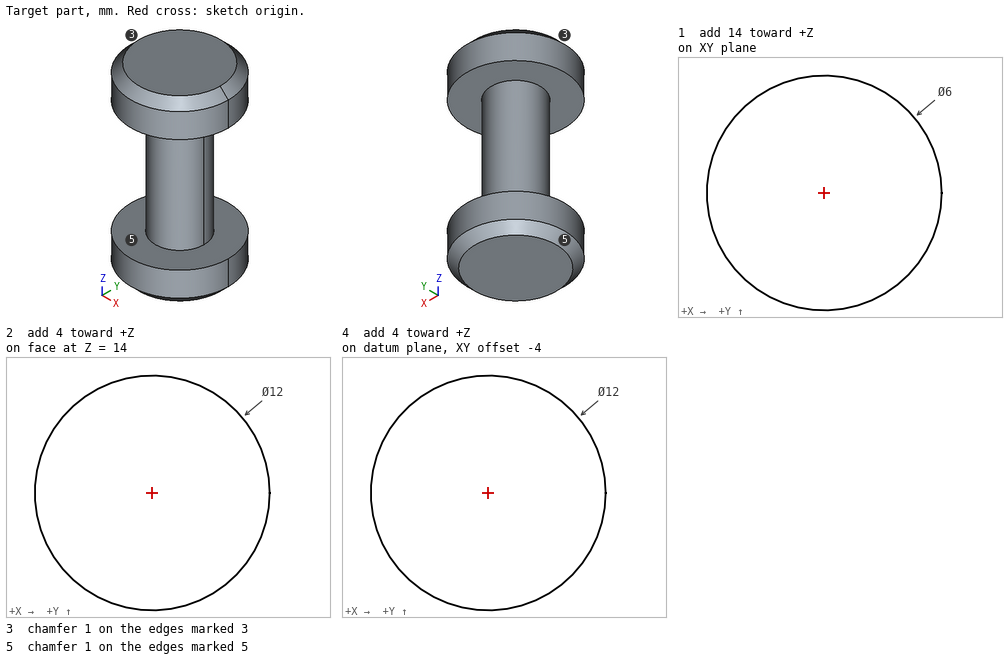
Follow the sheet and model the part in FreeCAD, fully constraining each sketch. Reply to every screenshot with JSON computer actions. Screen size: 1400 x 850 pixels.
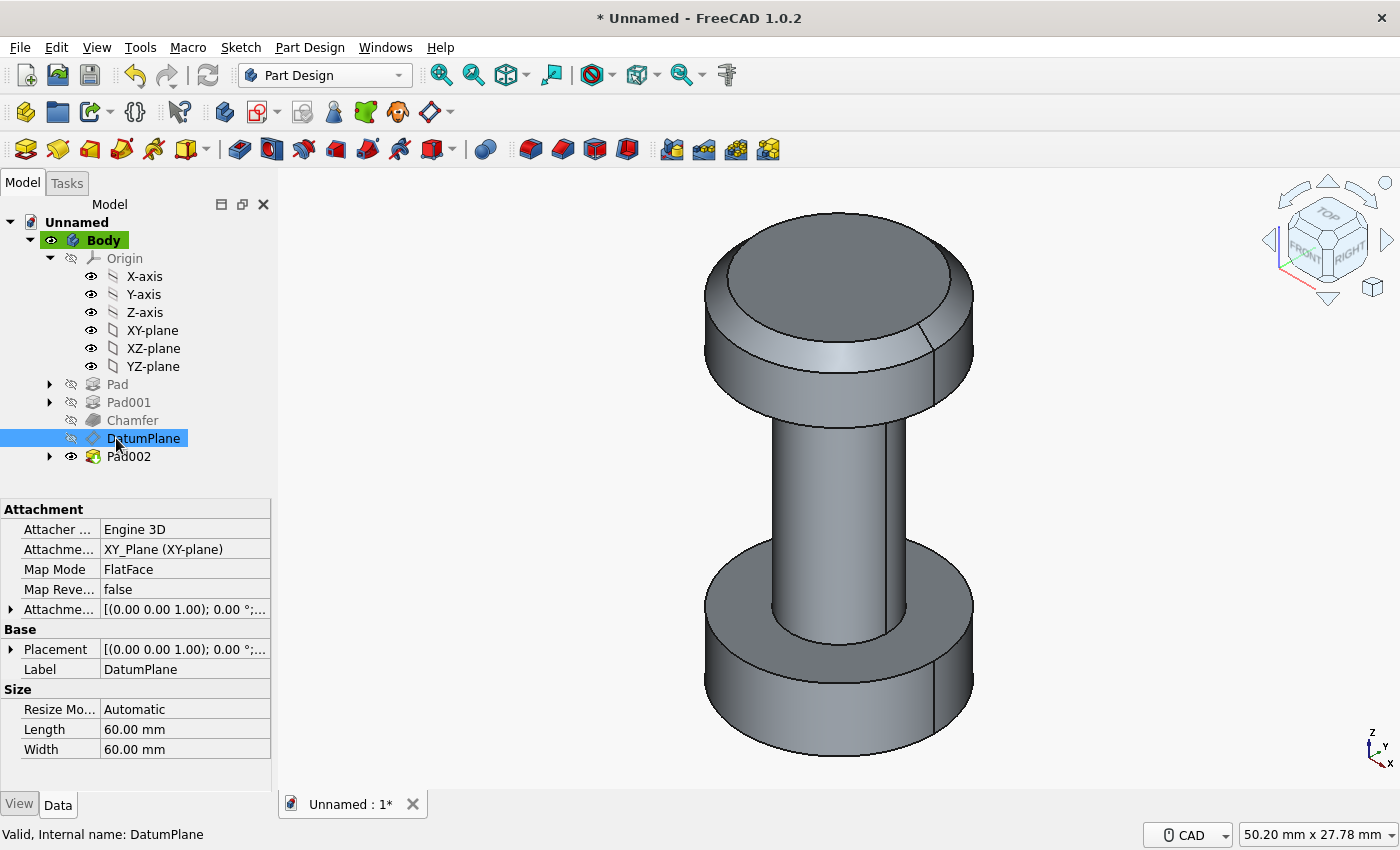
{"action": "key", "text": "2"}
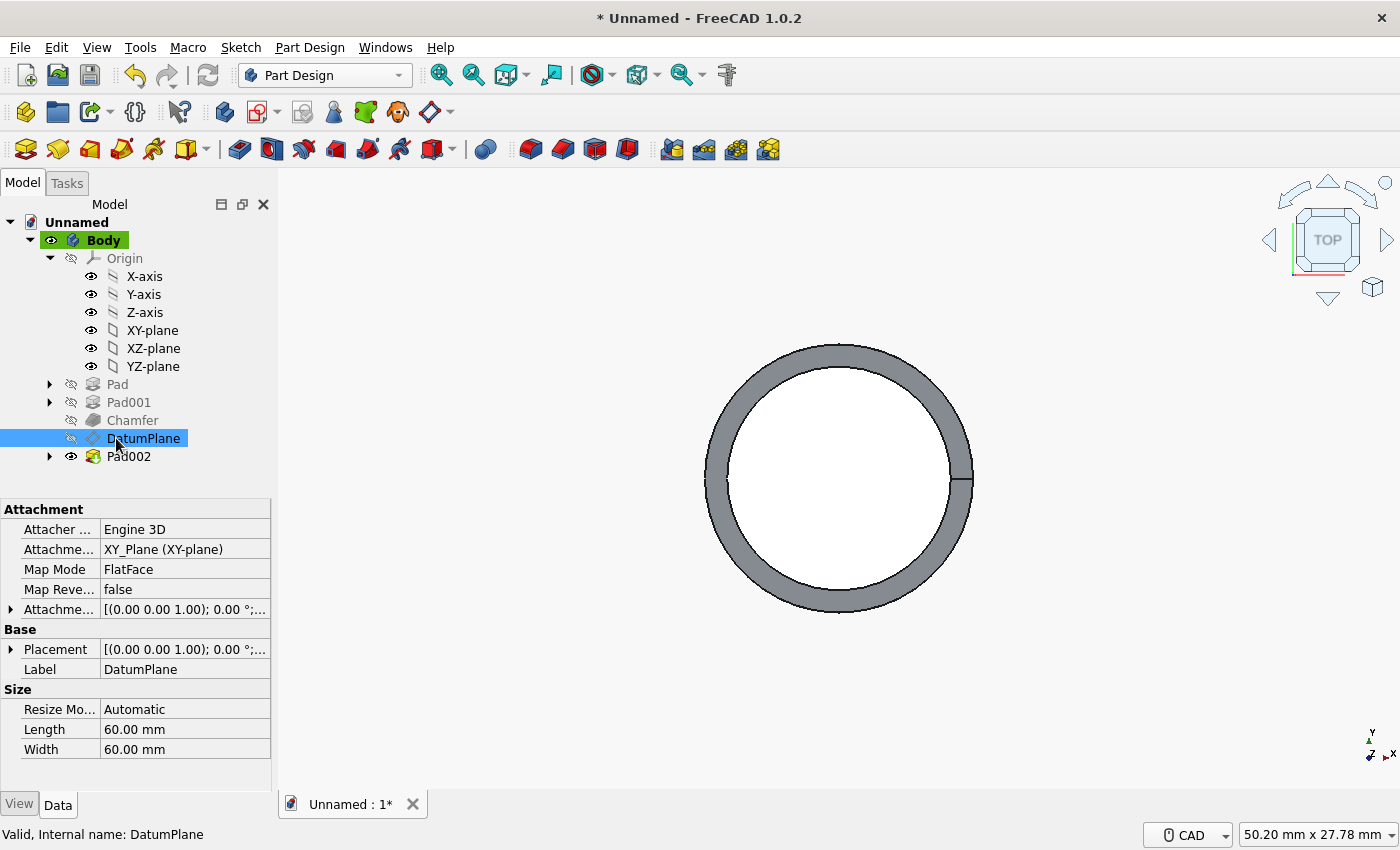
{"action": "key", "text": "v f"}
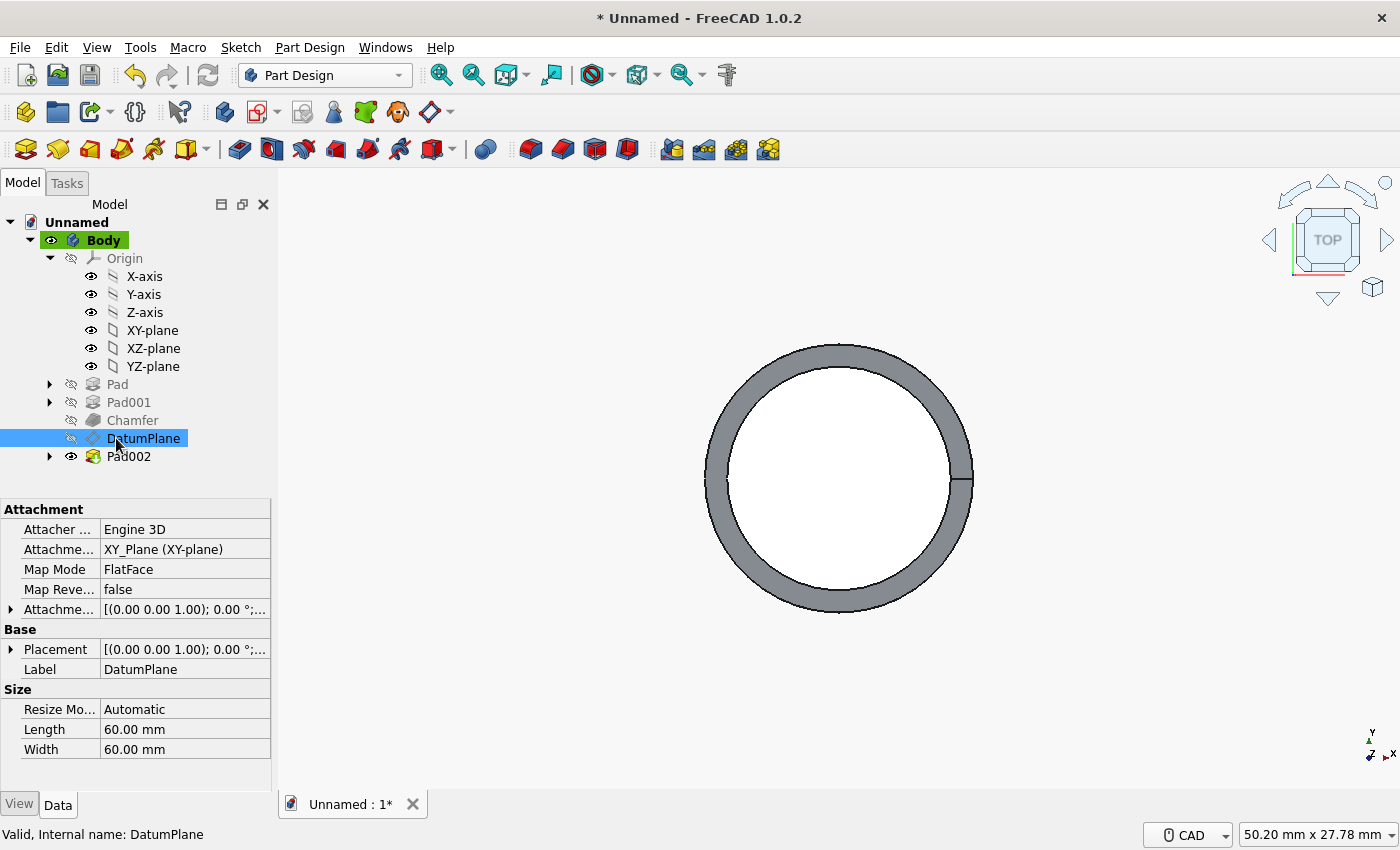
{"action": "key", "text": "1"}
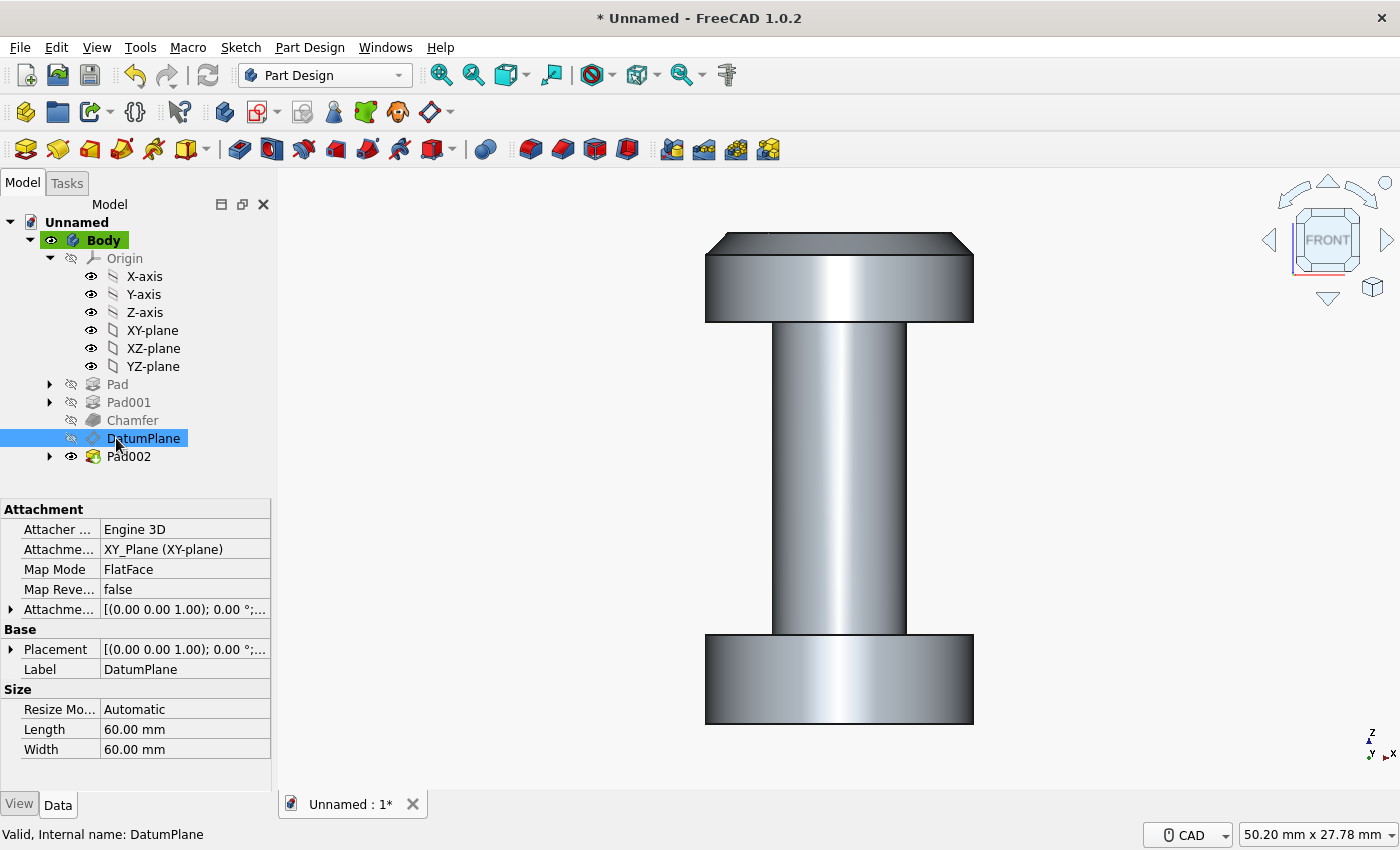
{"action": "left_click", "coordinate": [731, 723]}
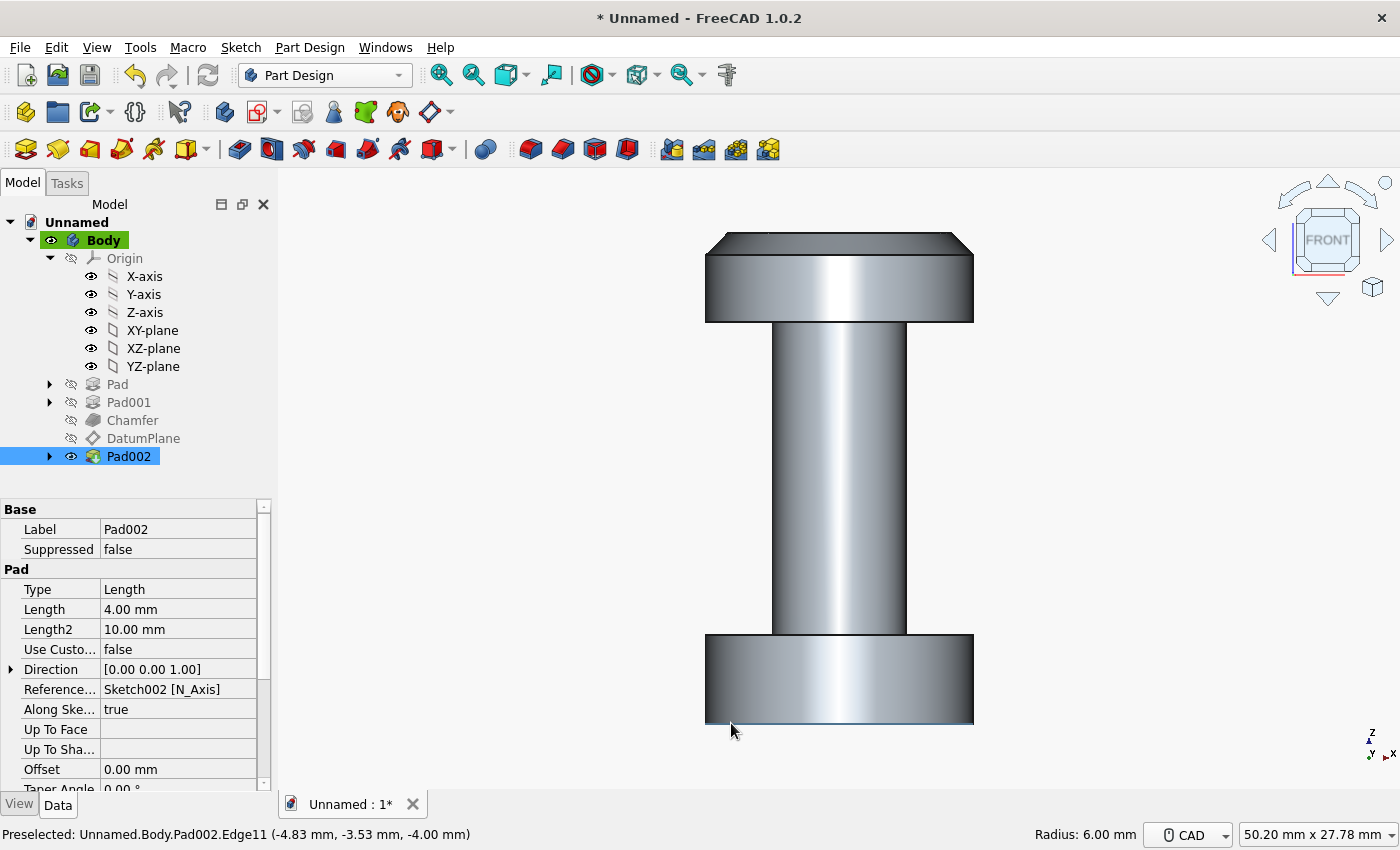
{"action": "left_click", "coordinate": [564, 150]}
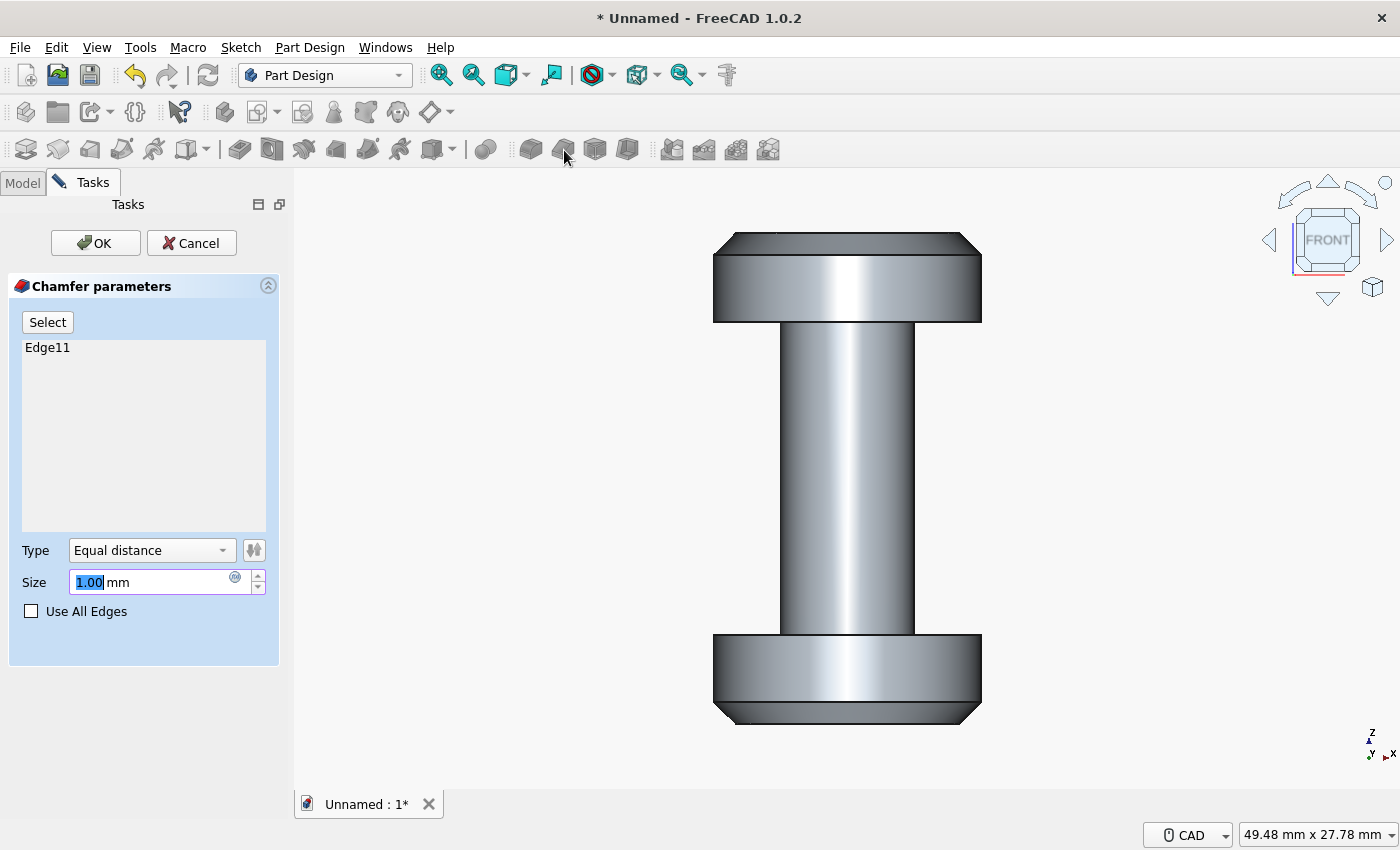
{"action": "type", "text": "1"}
{"action": "key", "text": "Tab"}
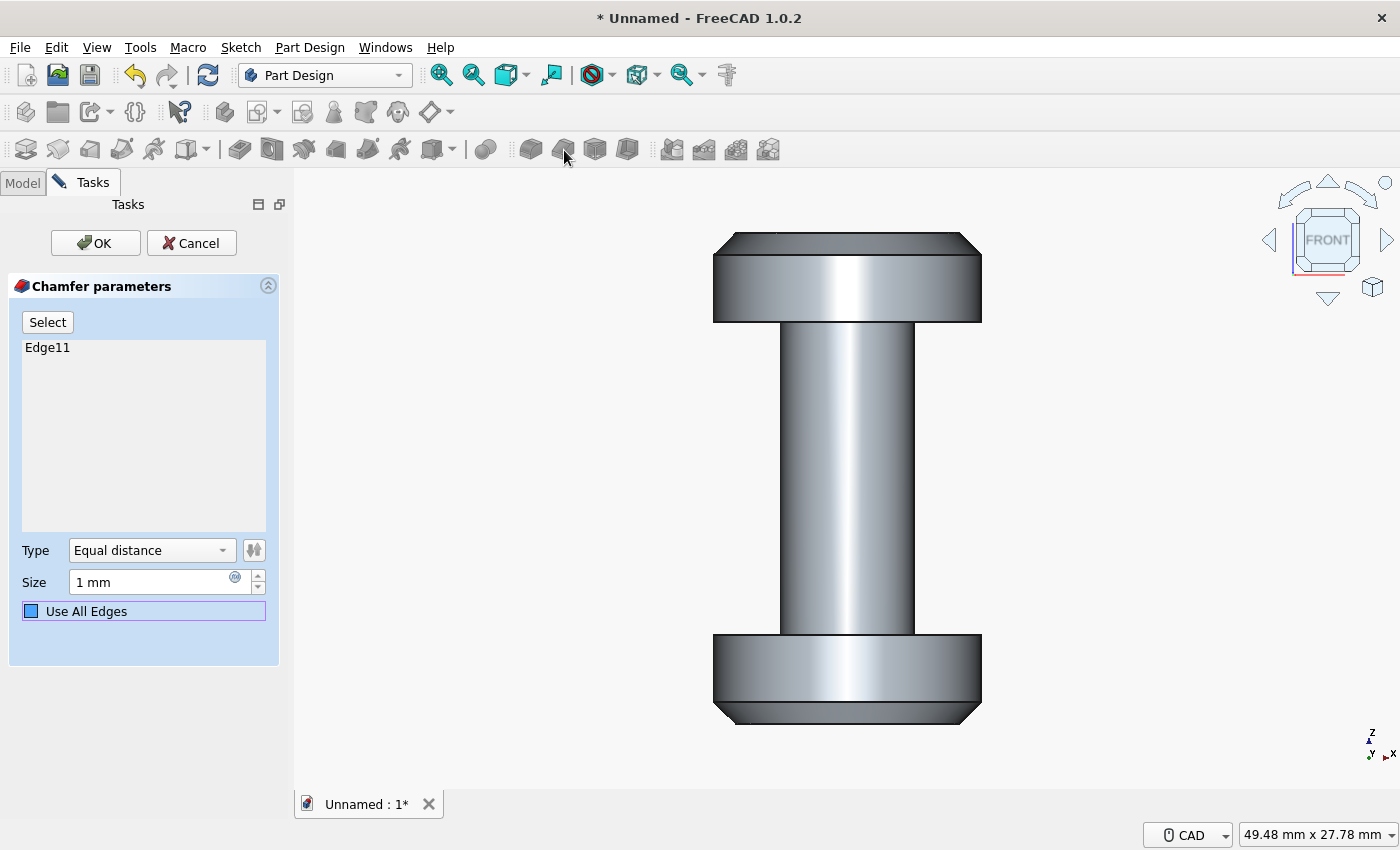
{"action": "left_click", "coordinate": [96, 243]}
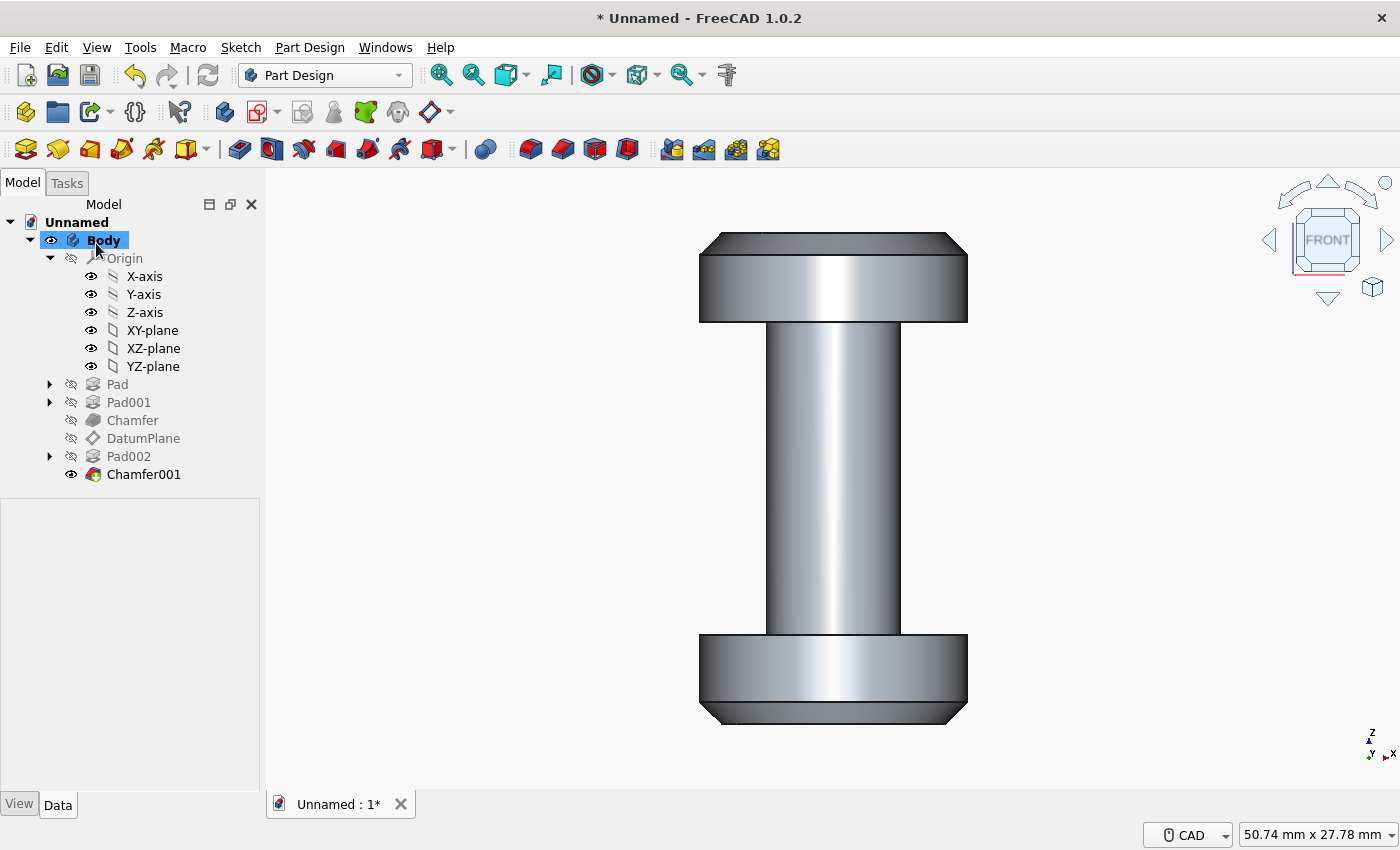
{"action": "key", "text": "0"}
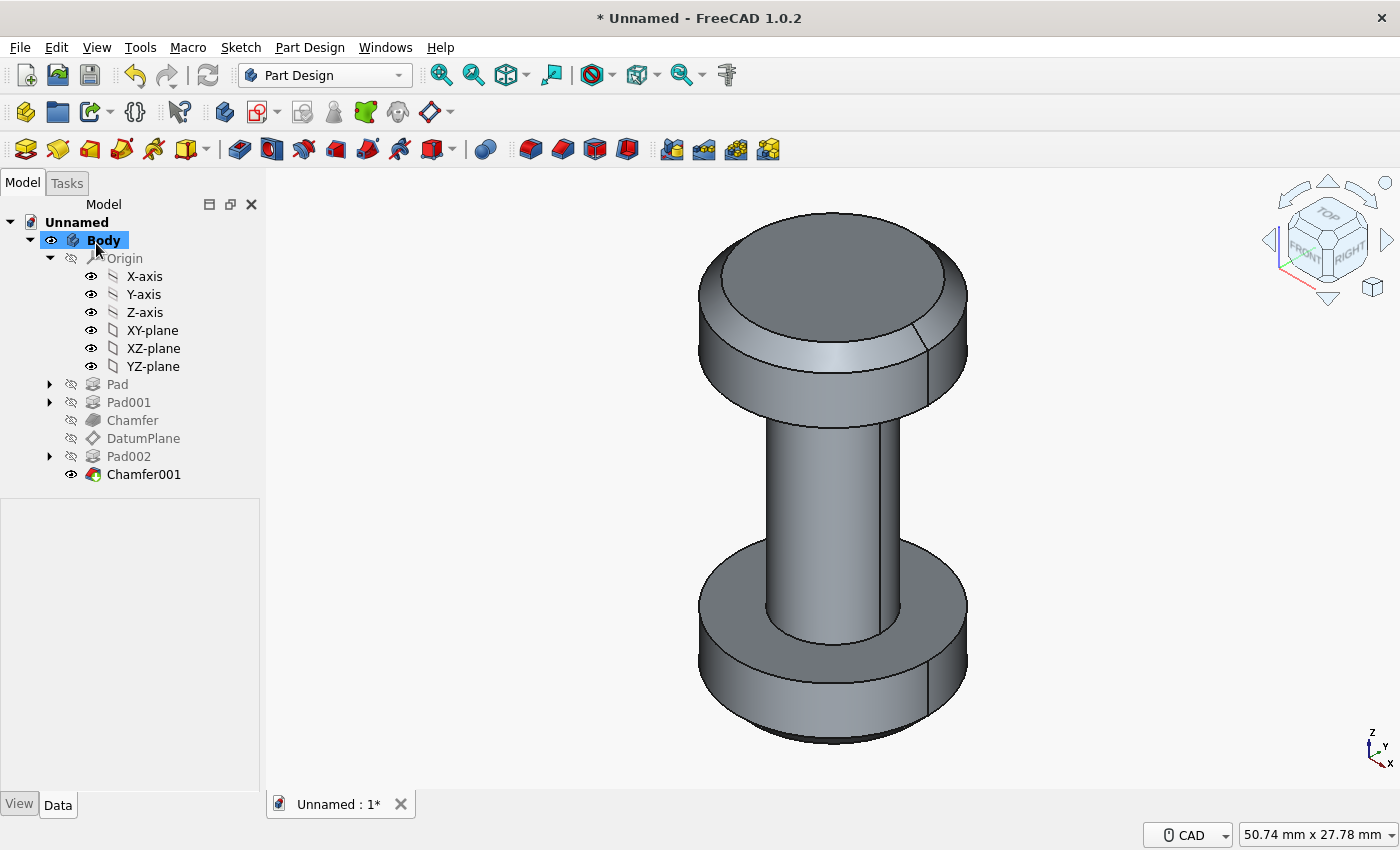
{"action": "key", "text": "v f"}